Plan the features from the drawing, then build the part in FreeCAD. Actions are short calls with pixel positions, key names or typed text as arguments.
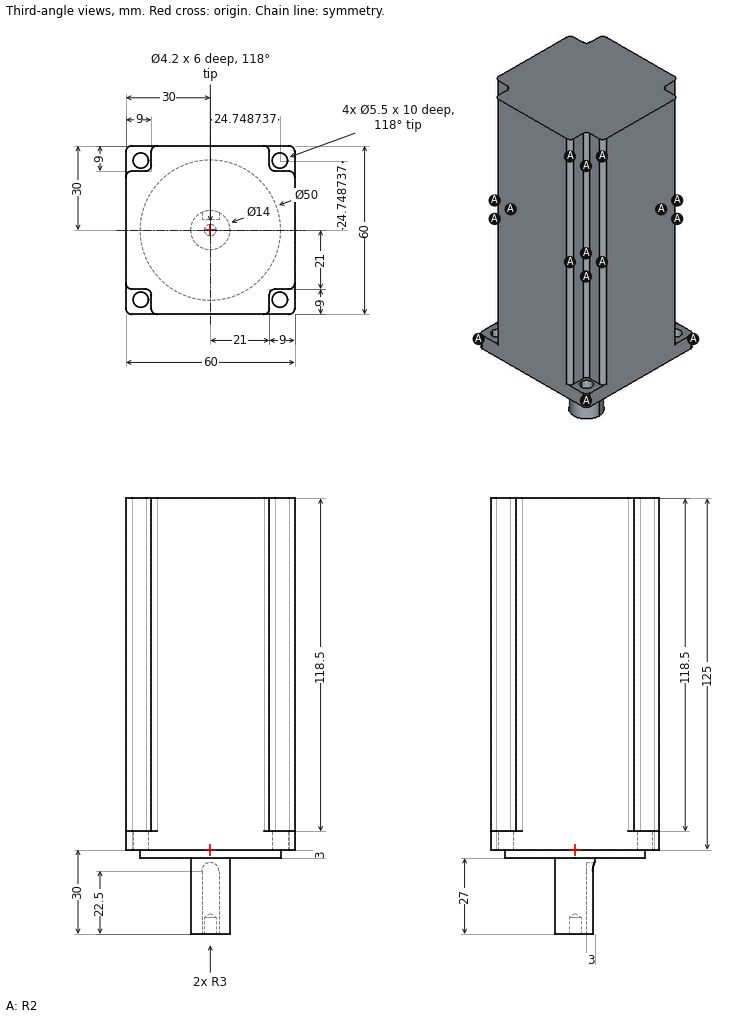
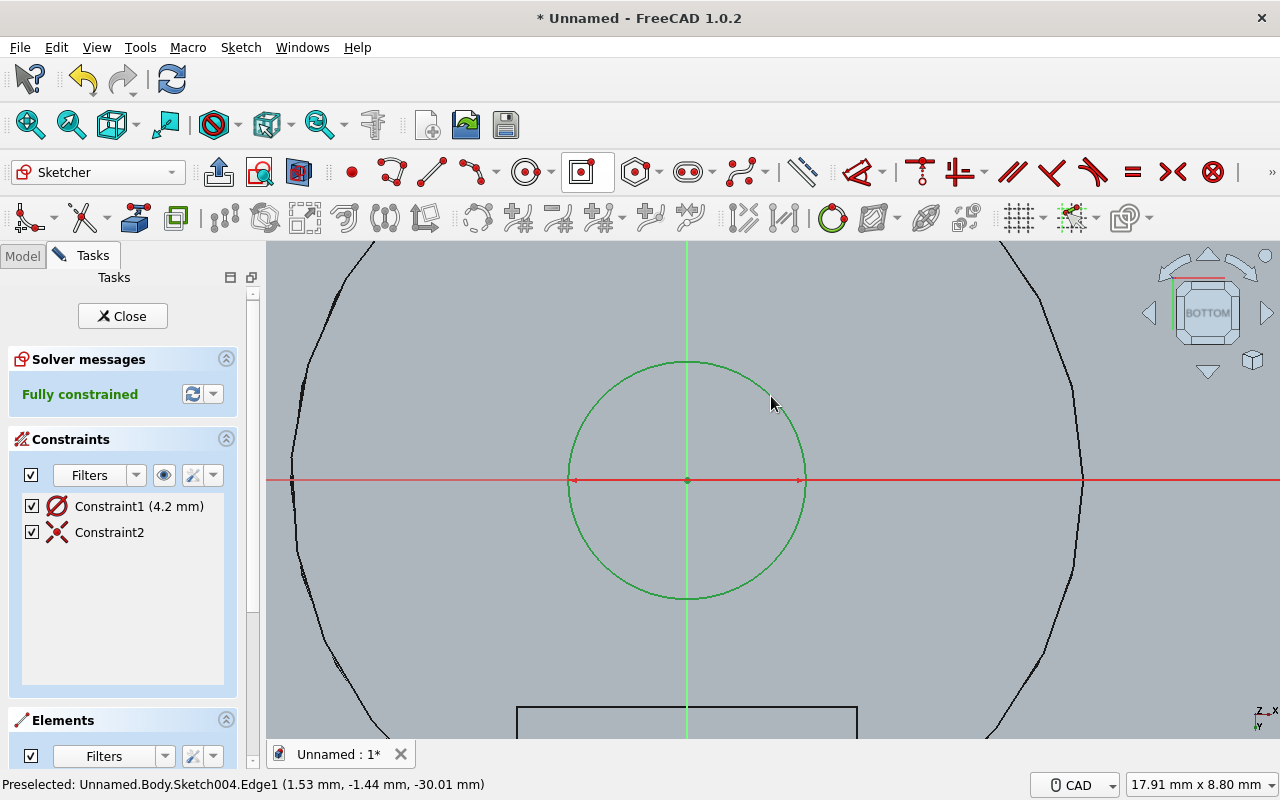
click(123, 316)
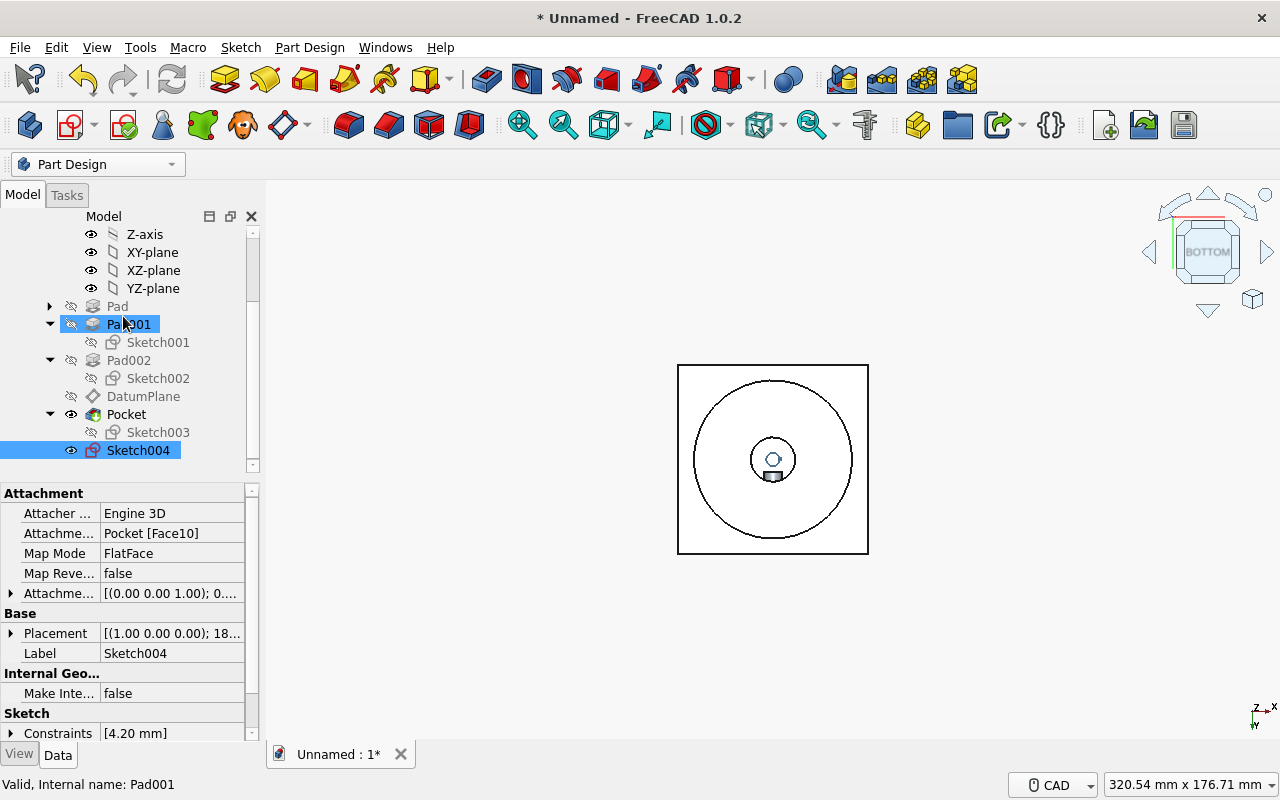
click(528, 80)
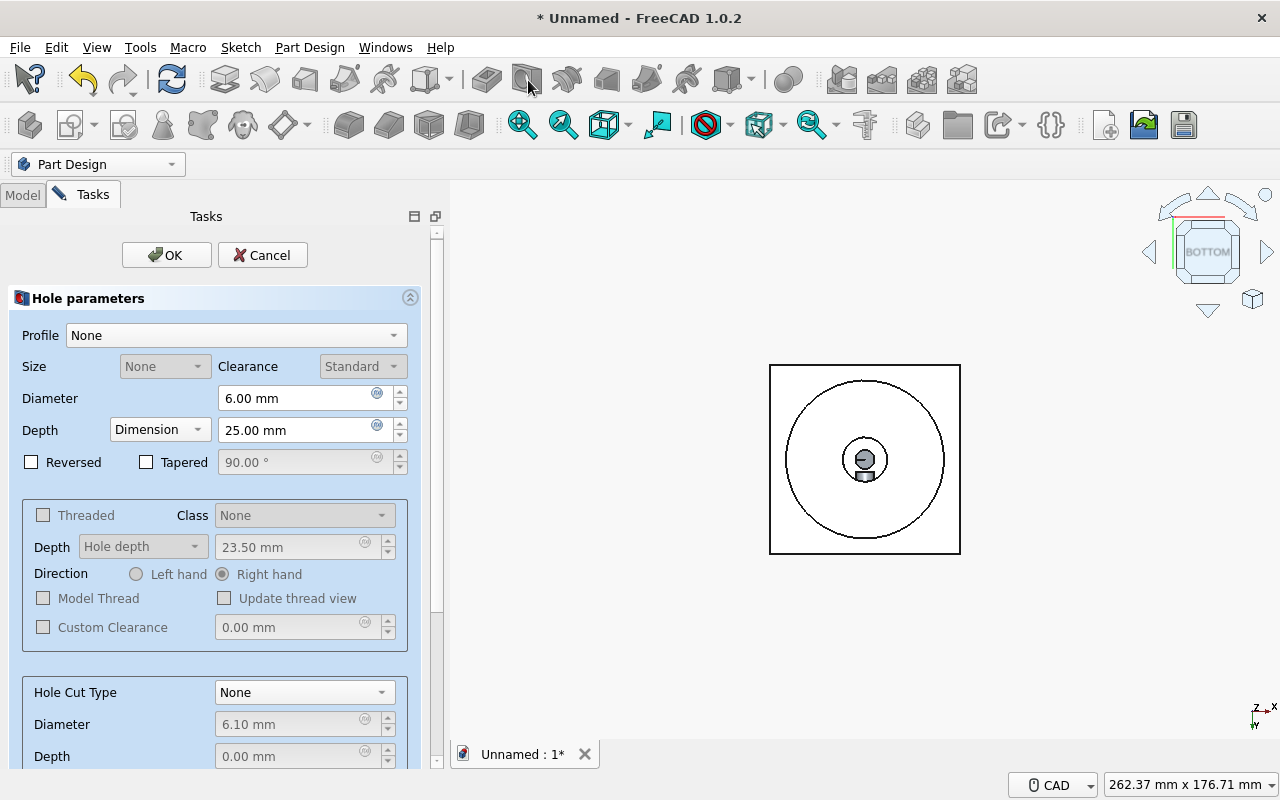
triple_click(305, 398)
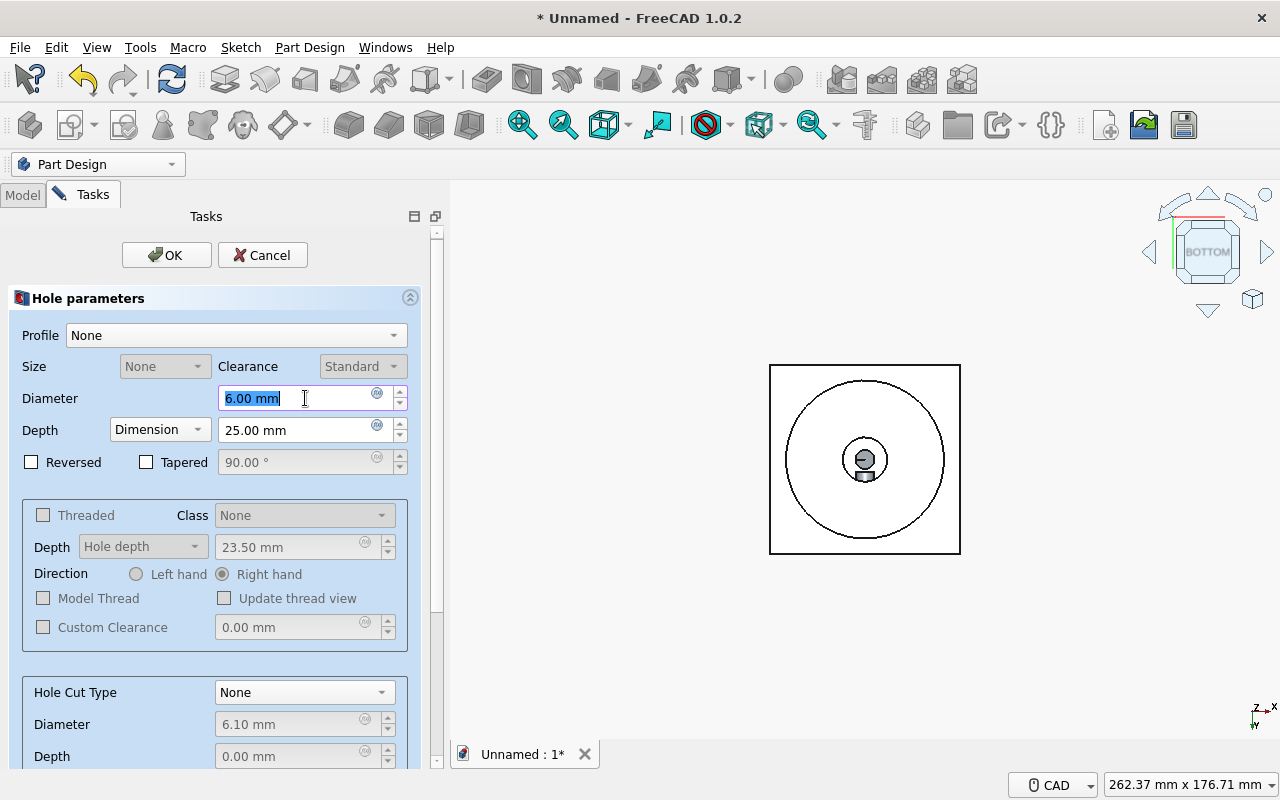
text(4.2)
key(Tab)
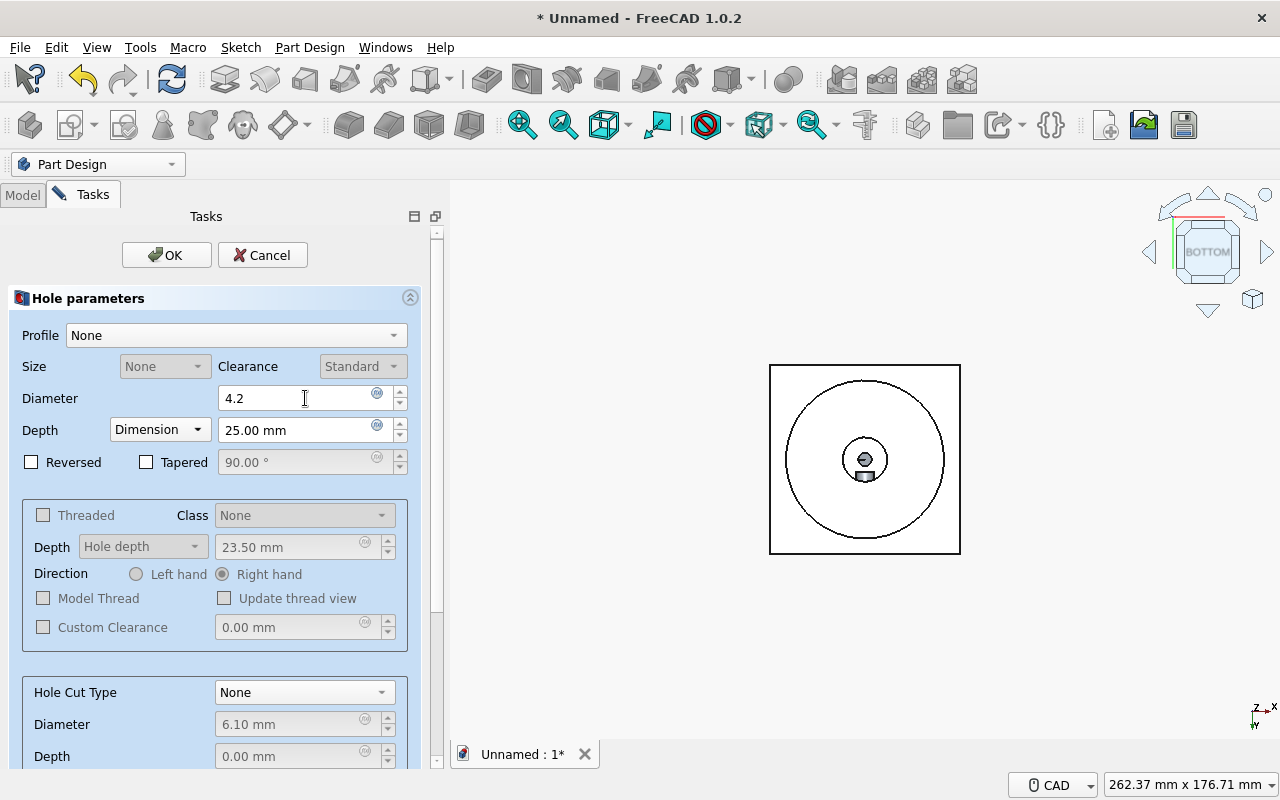
triple_click(305, 430)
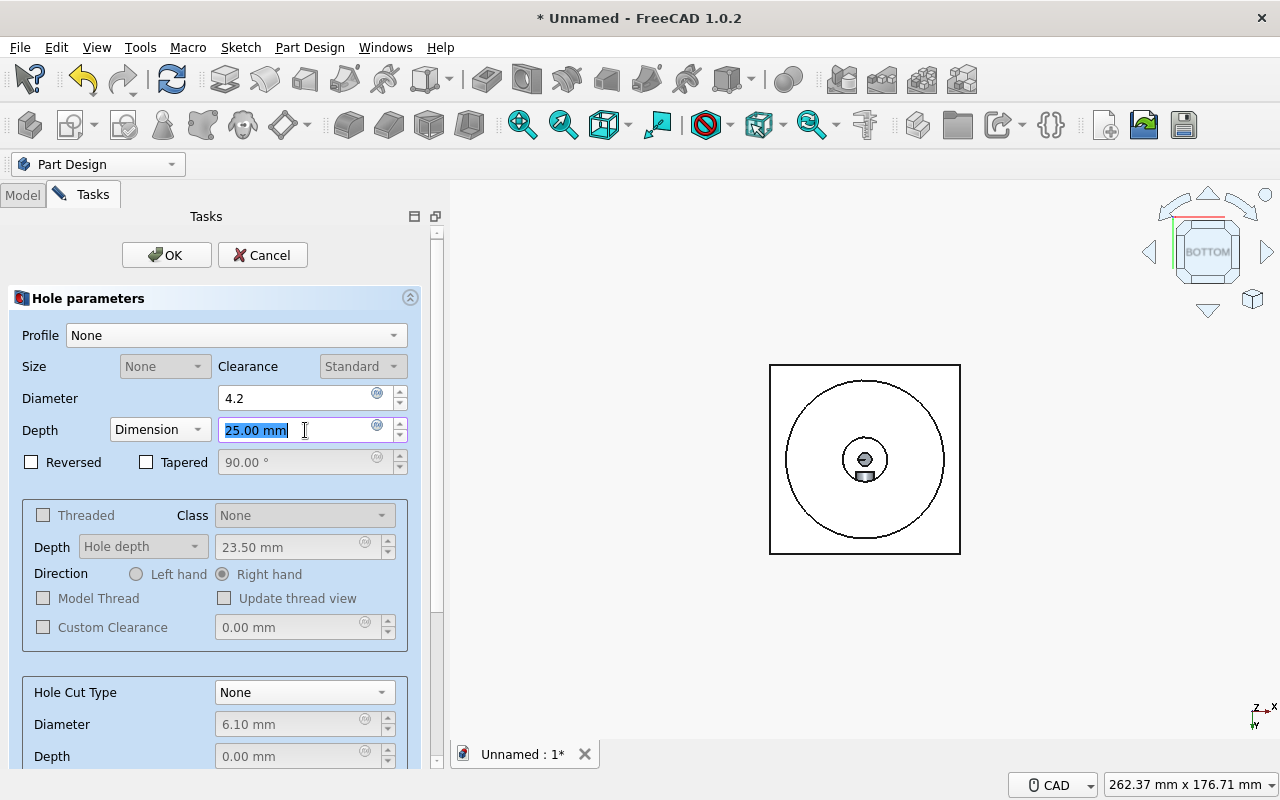
text(6)
key(Tab)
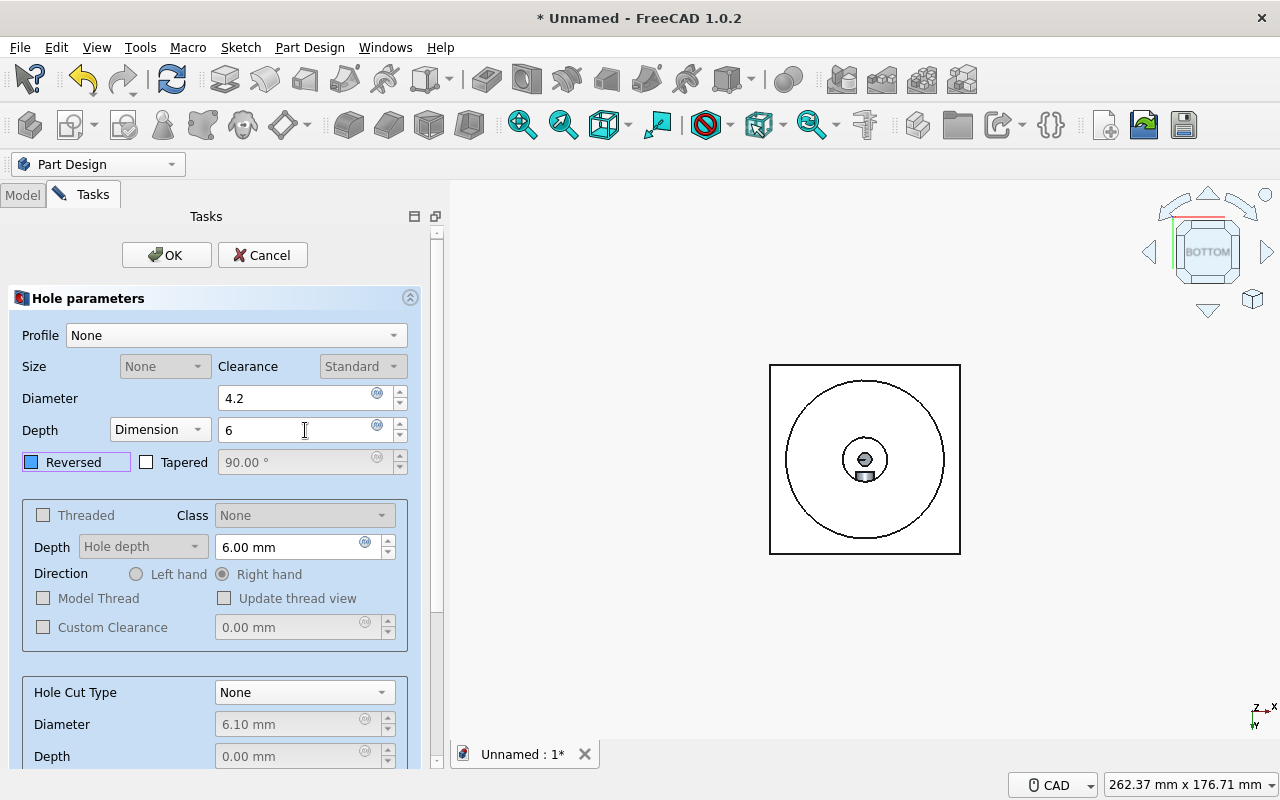
click(167, 255)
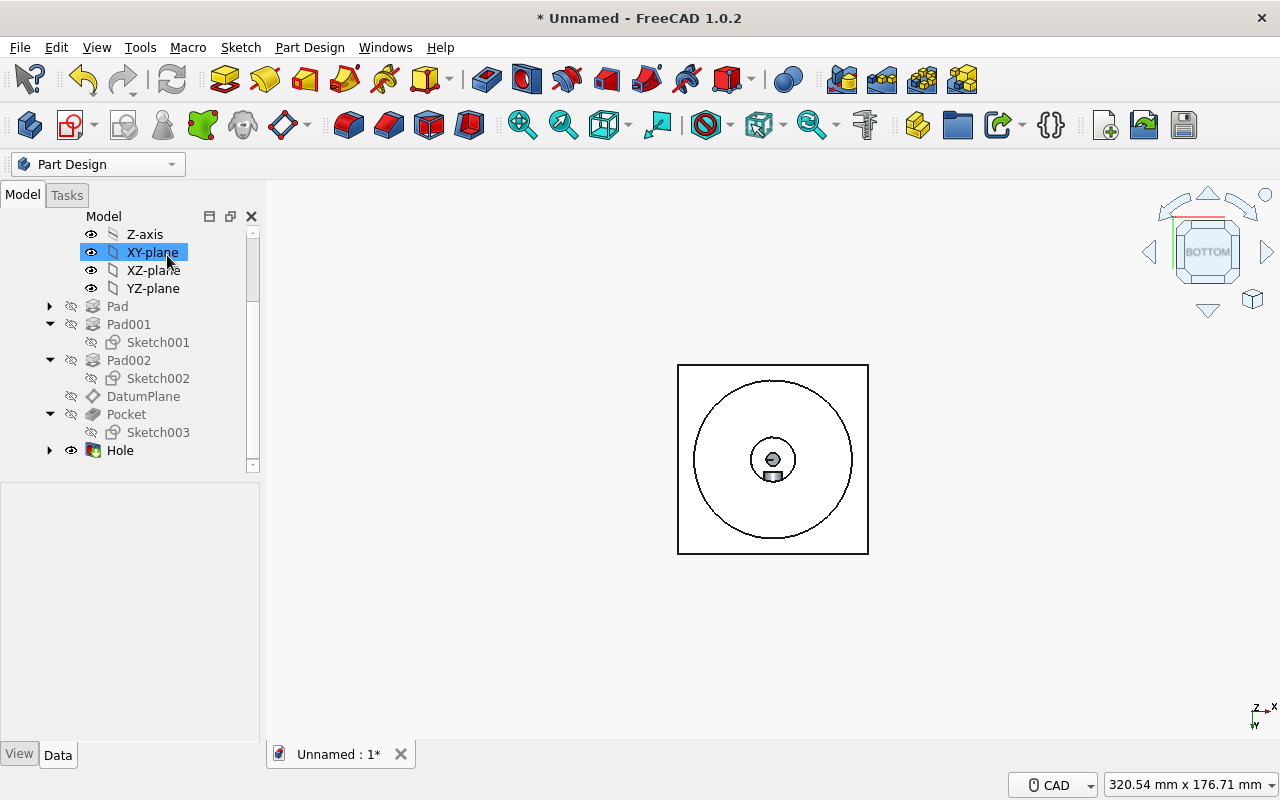
click(524, 126)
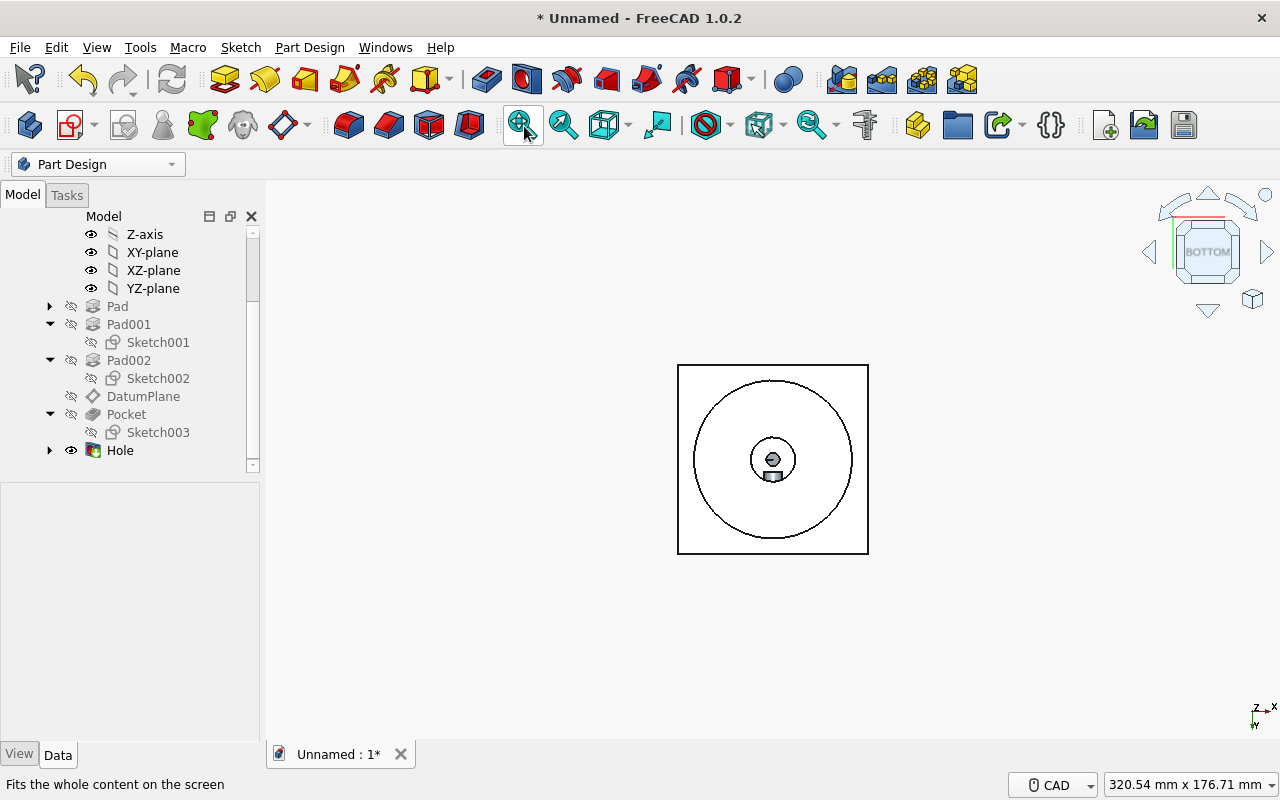
click(854, 540)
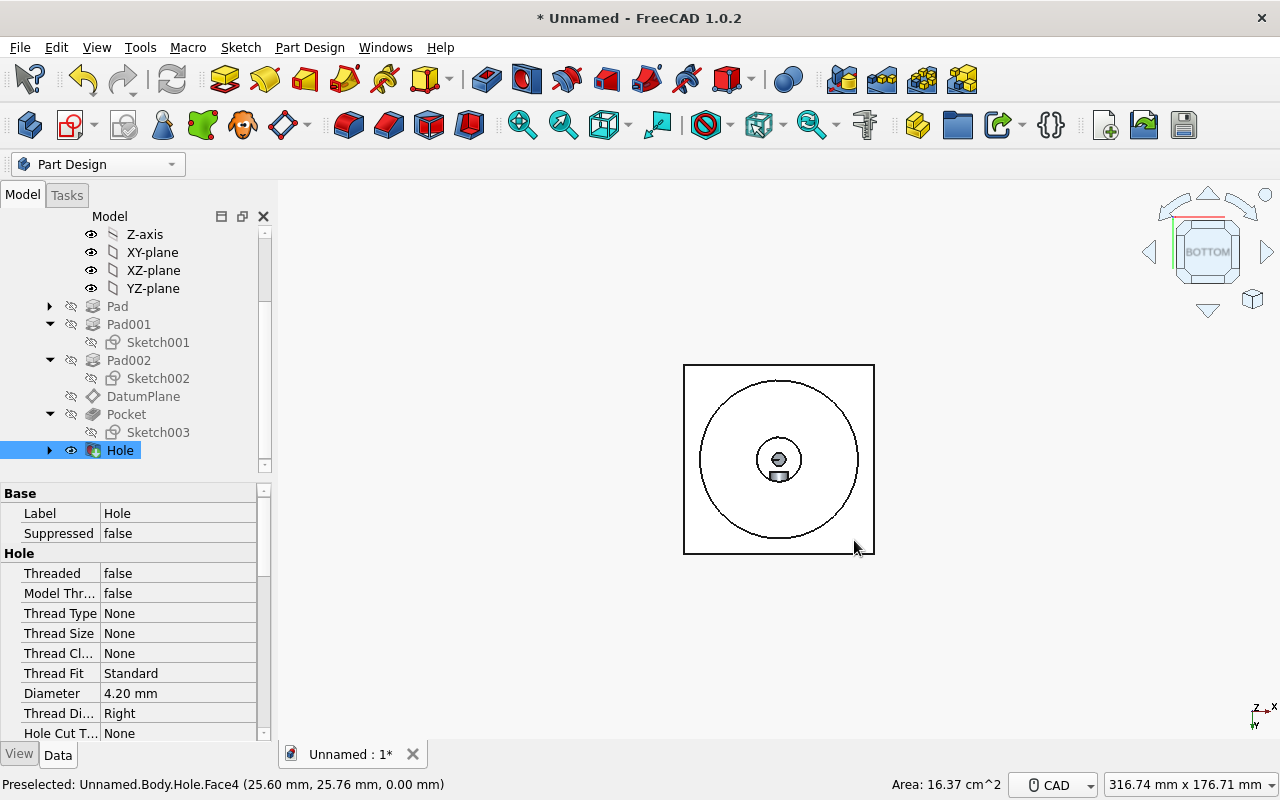
click(70, 126)